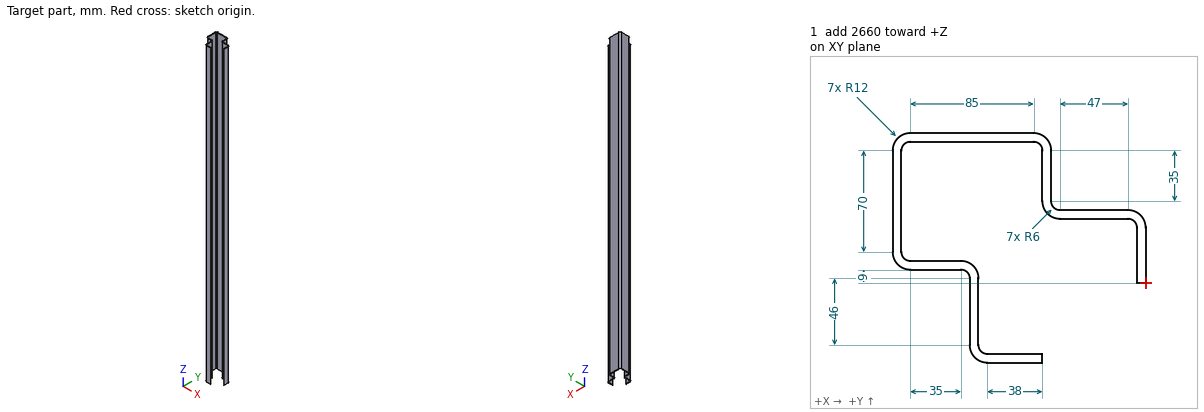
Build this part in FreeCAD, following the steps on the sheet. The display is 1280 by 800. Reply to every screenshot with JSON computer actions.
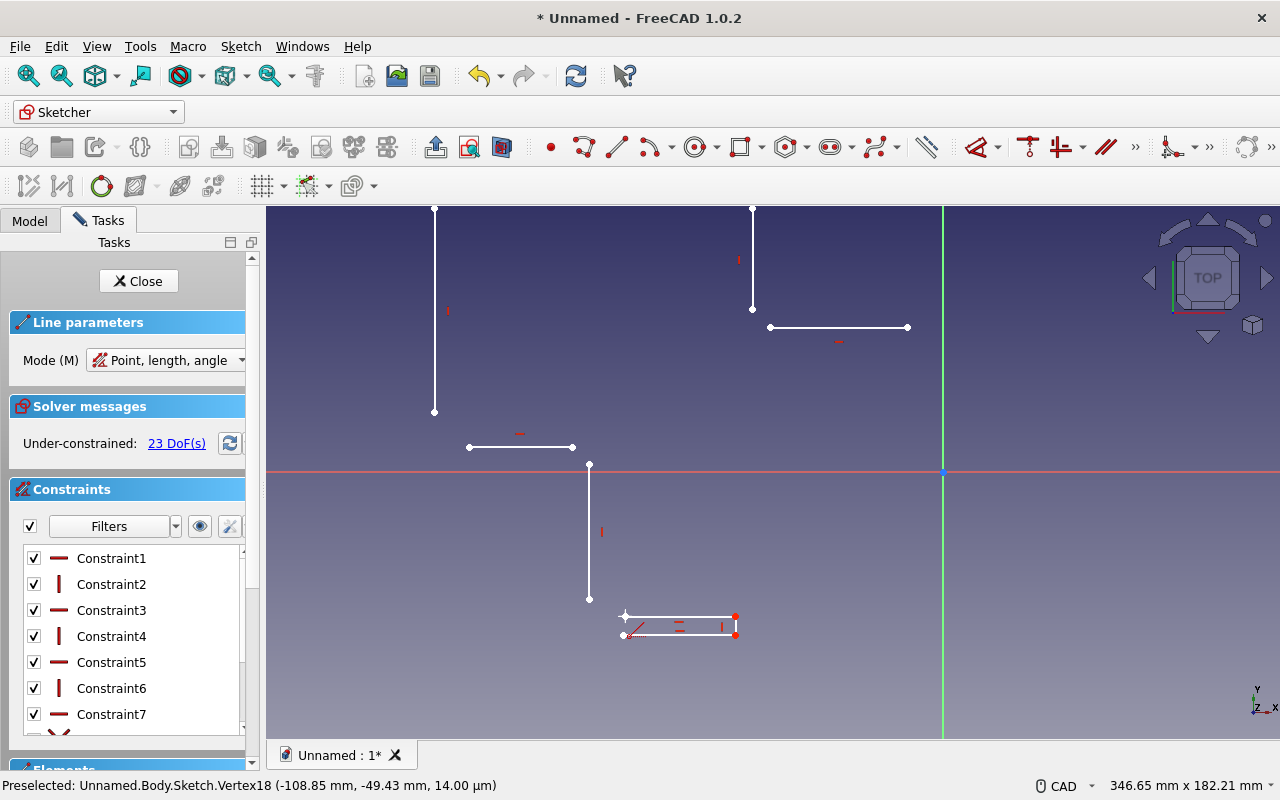
{"action": "left_click", "coordinate": [607, 598]}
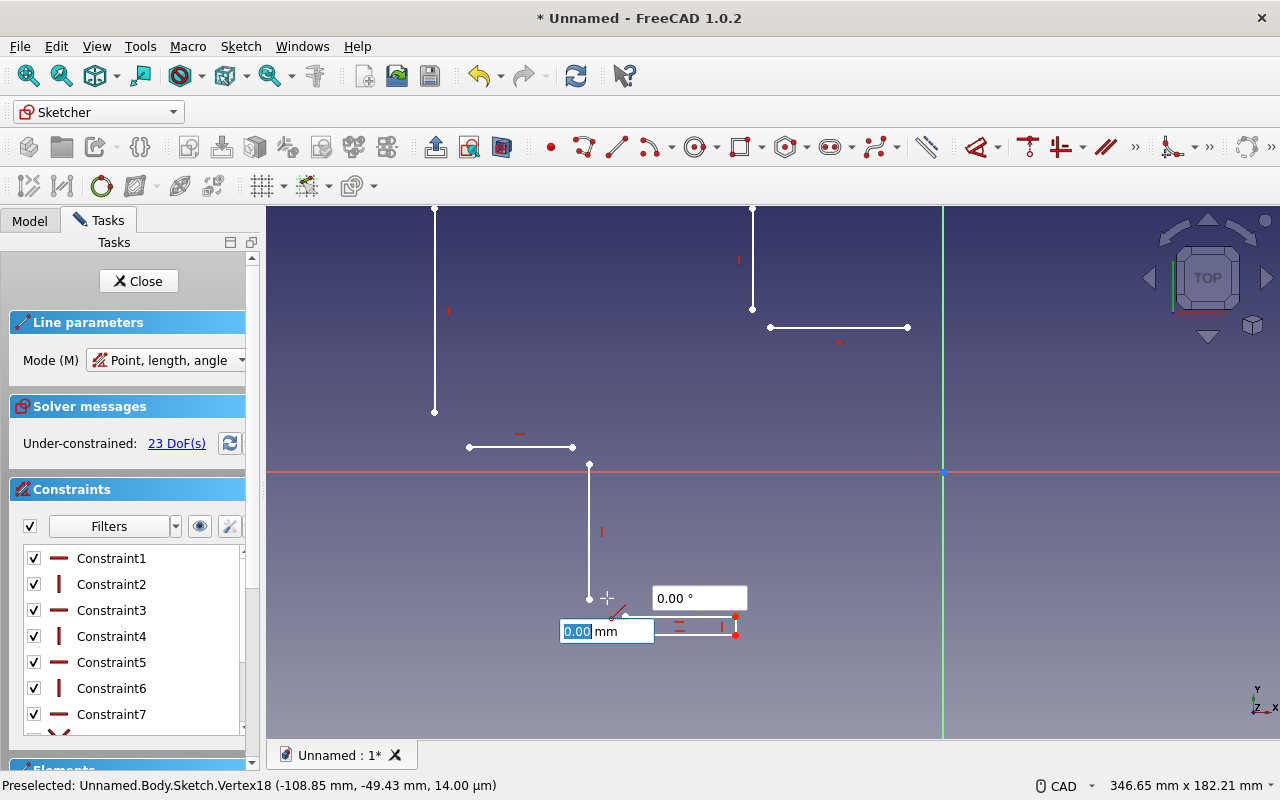
{"action": "scroll", "coordinate": [607, 464], "scroll_direction": "up", "scroll_amount": 3}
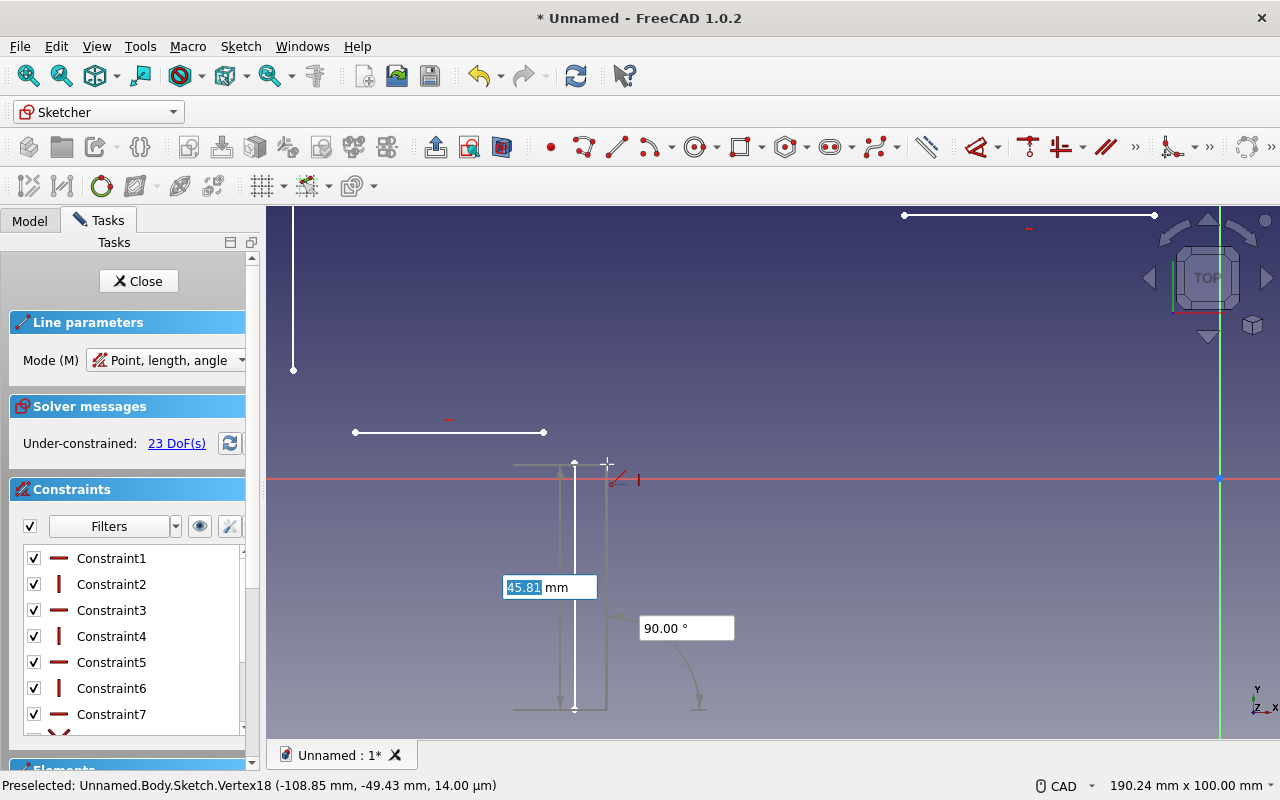
{"action": "left_click", "coordinate": [607, 463]}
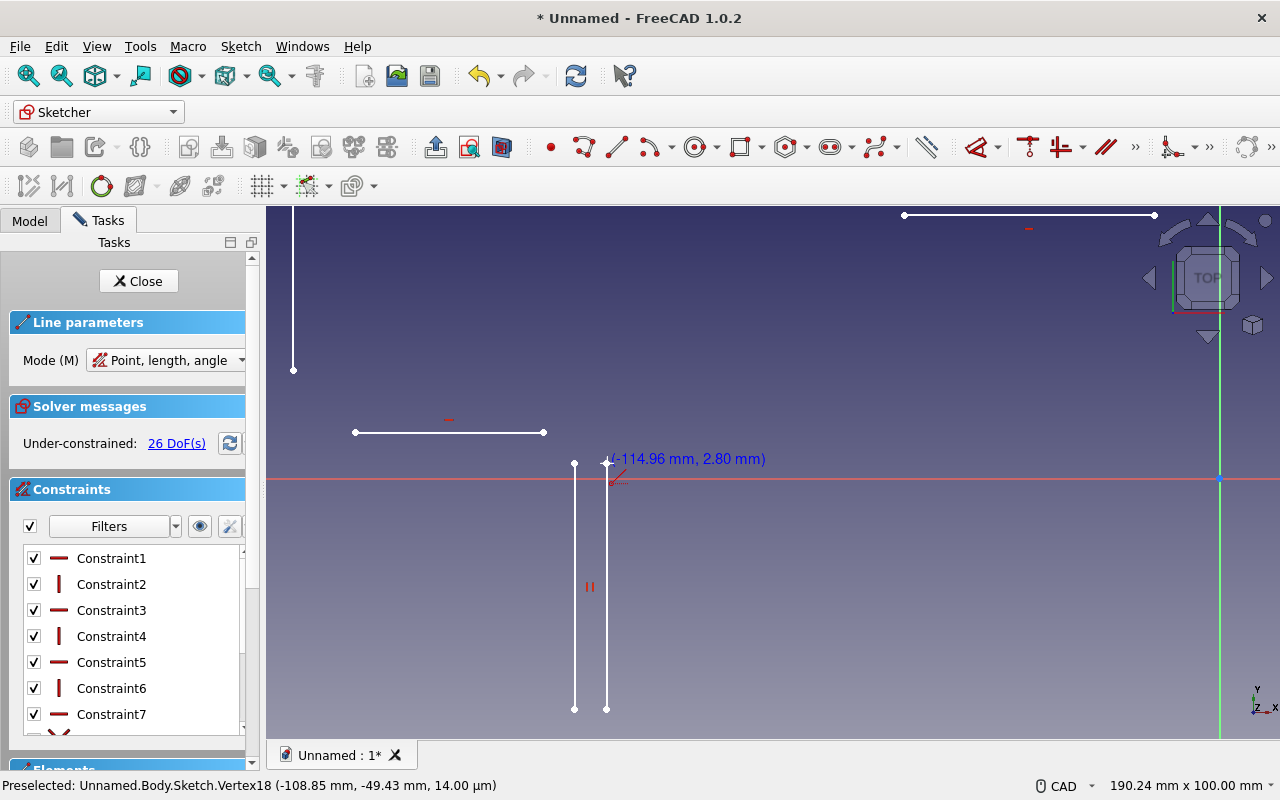
{"action": "left_click", "coordinate": [543, 399]}
{"action": "left_click", "coordinate": [356, 399]}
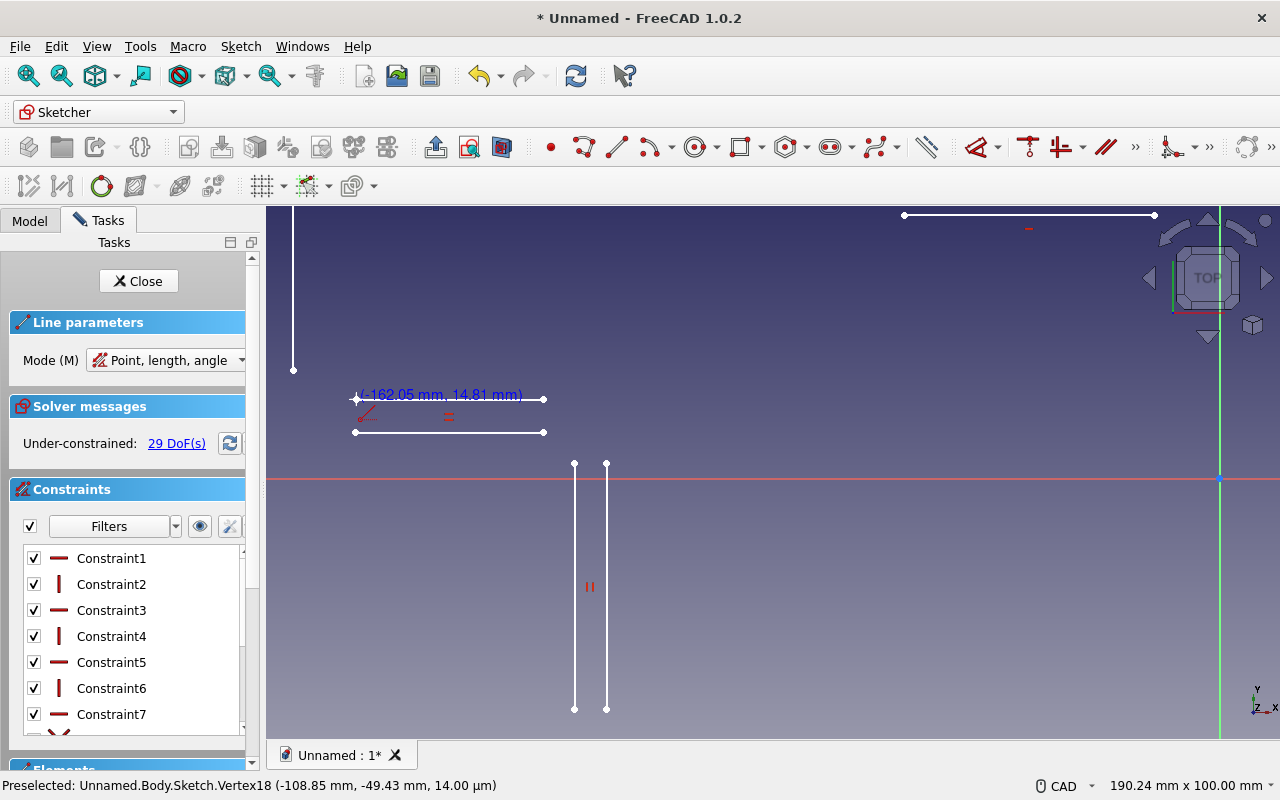
{"action": "left_click", "coordinate": [324, 367]}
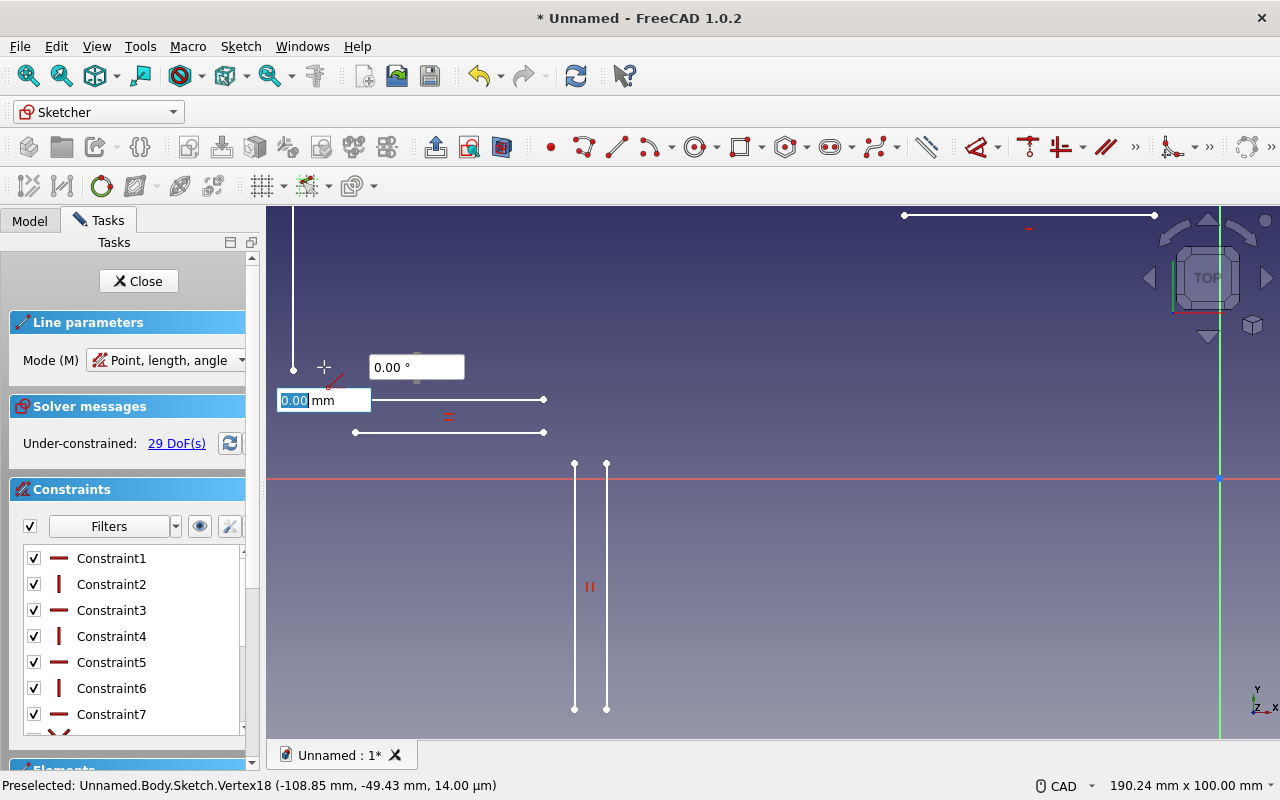
{"action": "scroll", "coordinate": [675, 543], "scroll_direction": "down", "scroll_amount": 5}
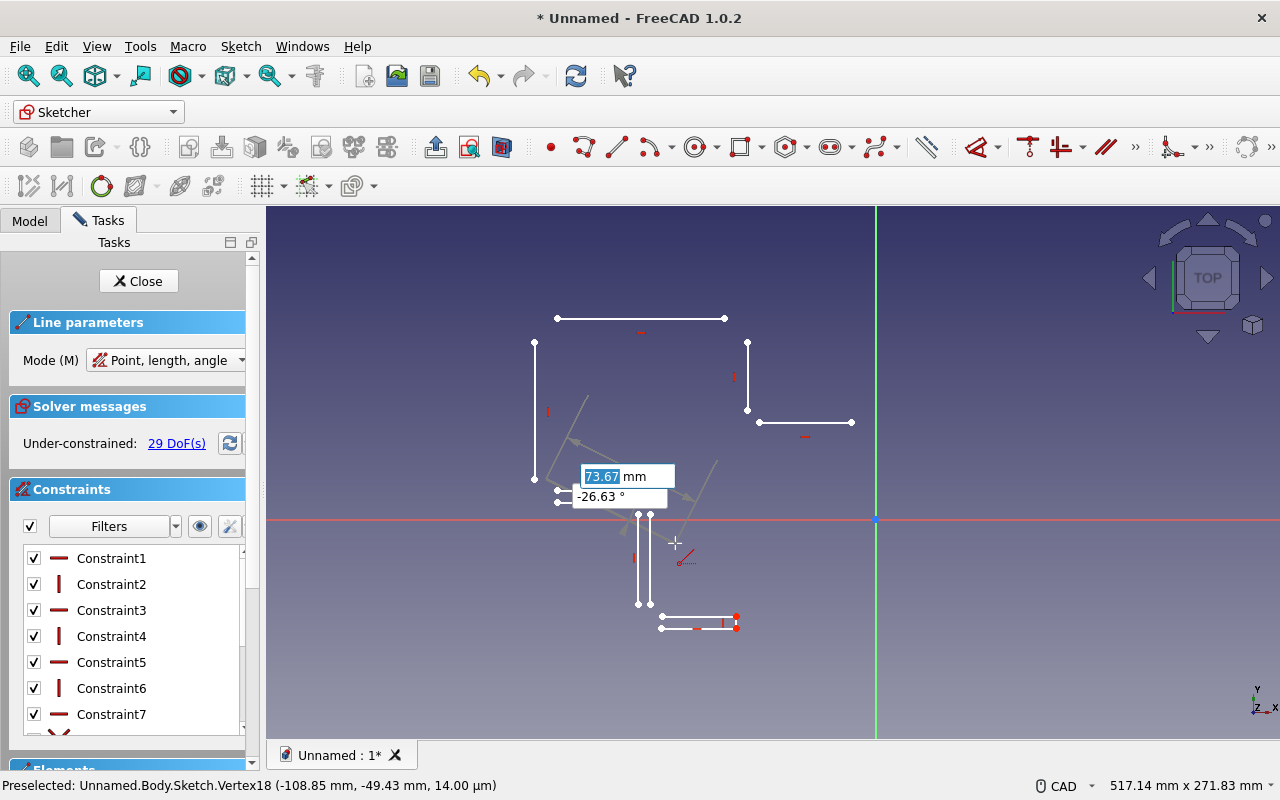
{"action": "scroll", "coordinate": [546, 341], "scroll_direction": "up", "scroll_amount": 2}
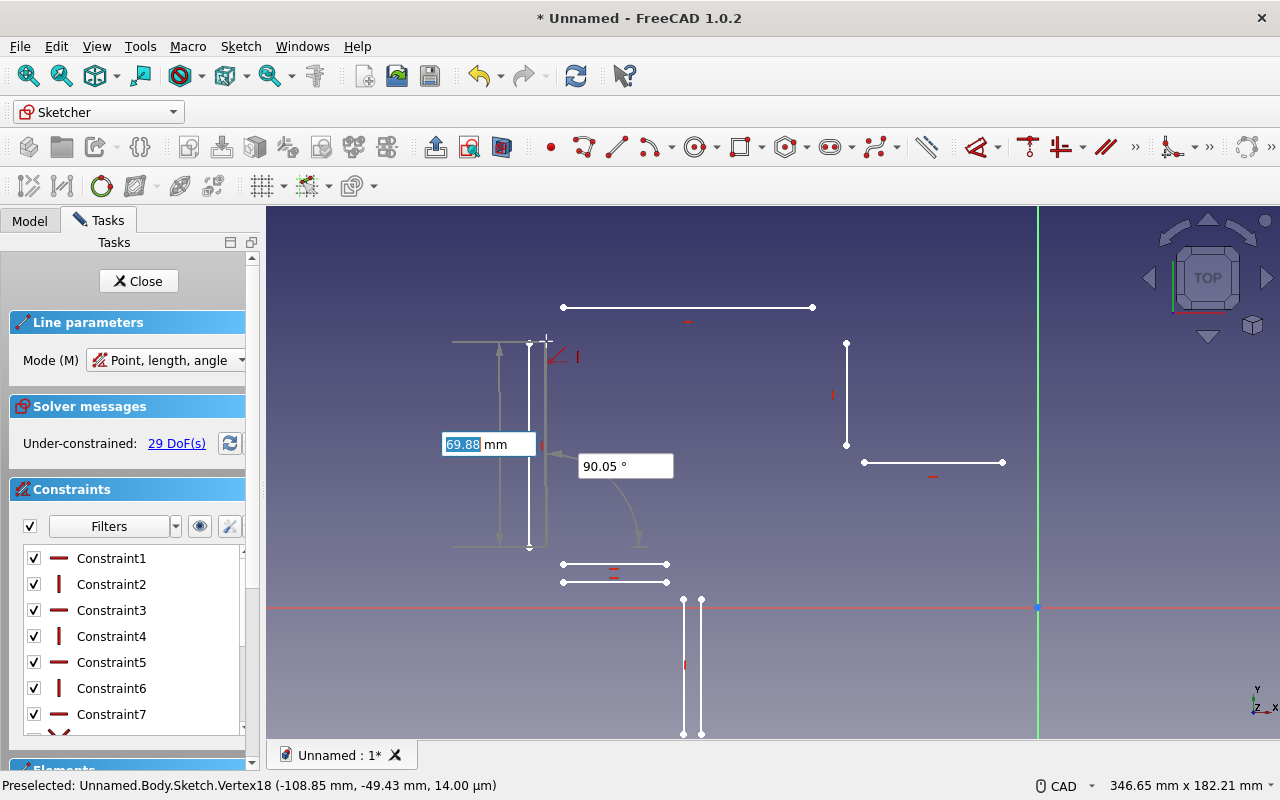
{"action": "left_click", "coordinate": [546, 341]}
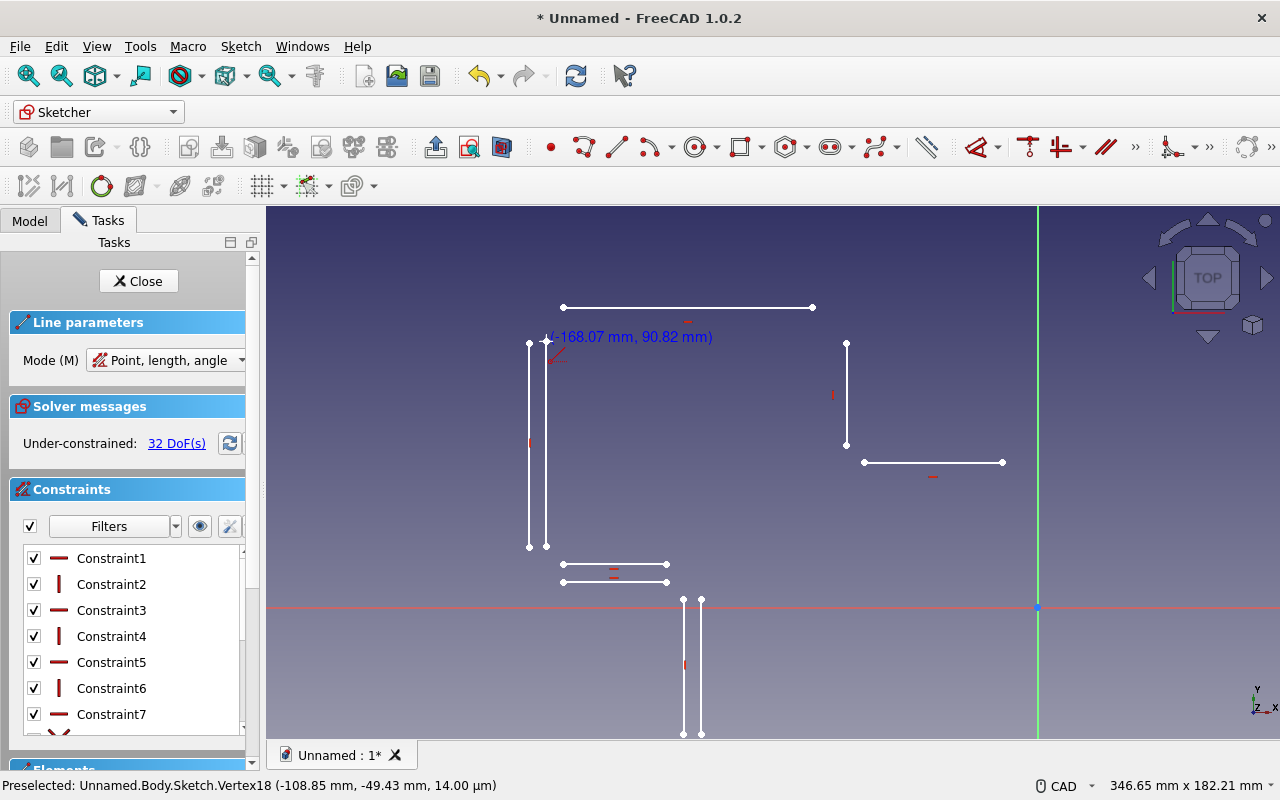
{"action": "left_click", "coordinate": [564, 324]}
{"action": "left_click", "coordinate": [812, 324]}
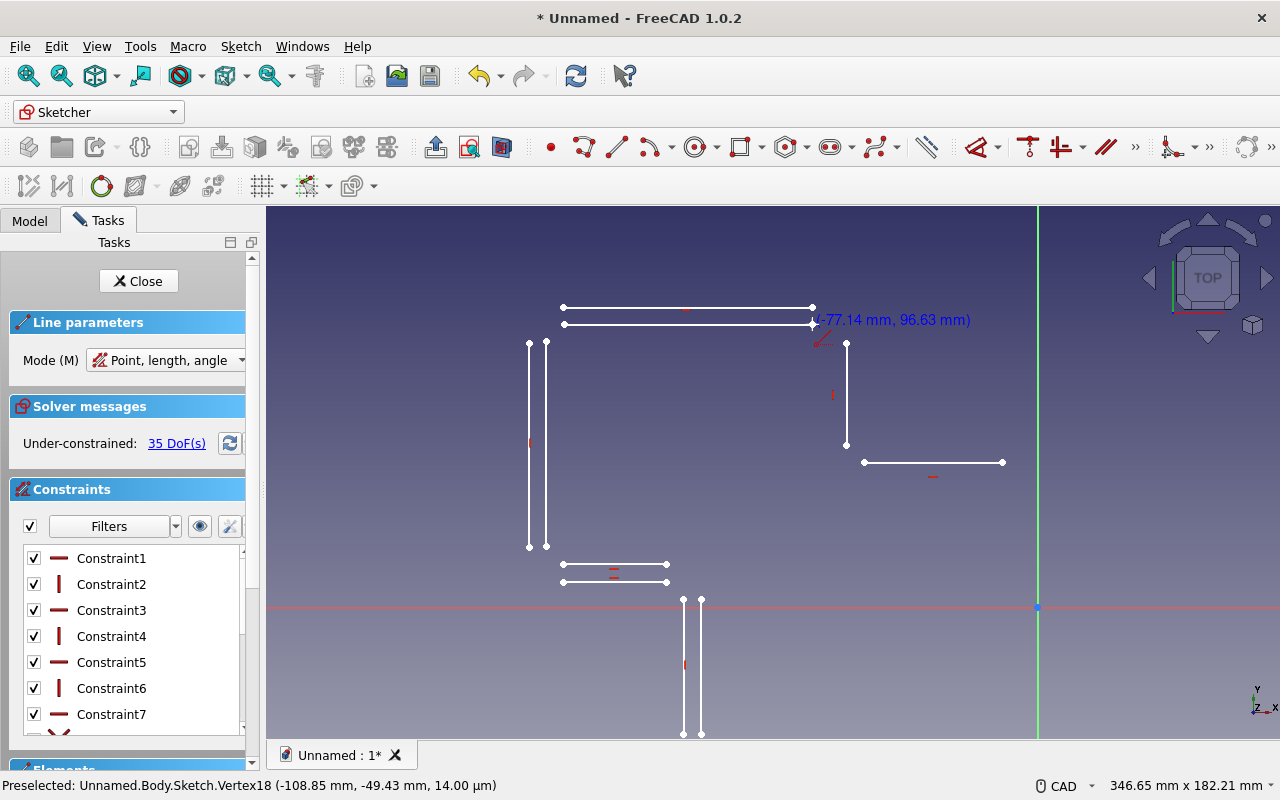
{"action": "left_click", "coordinate": [830, 341]}
{"action": "left_click", "coordinate": [830, 444]}